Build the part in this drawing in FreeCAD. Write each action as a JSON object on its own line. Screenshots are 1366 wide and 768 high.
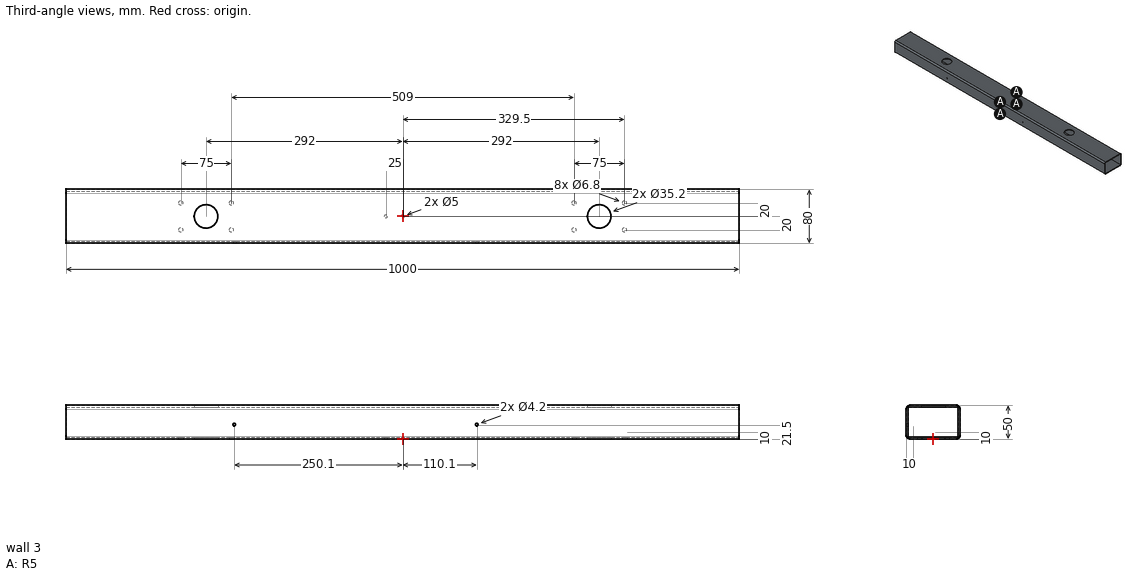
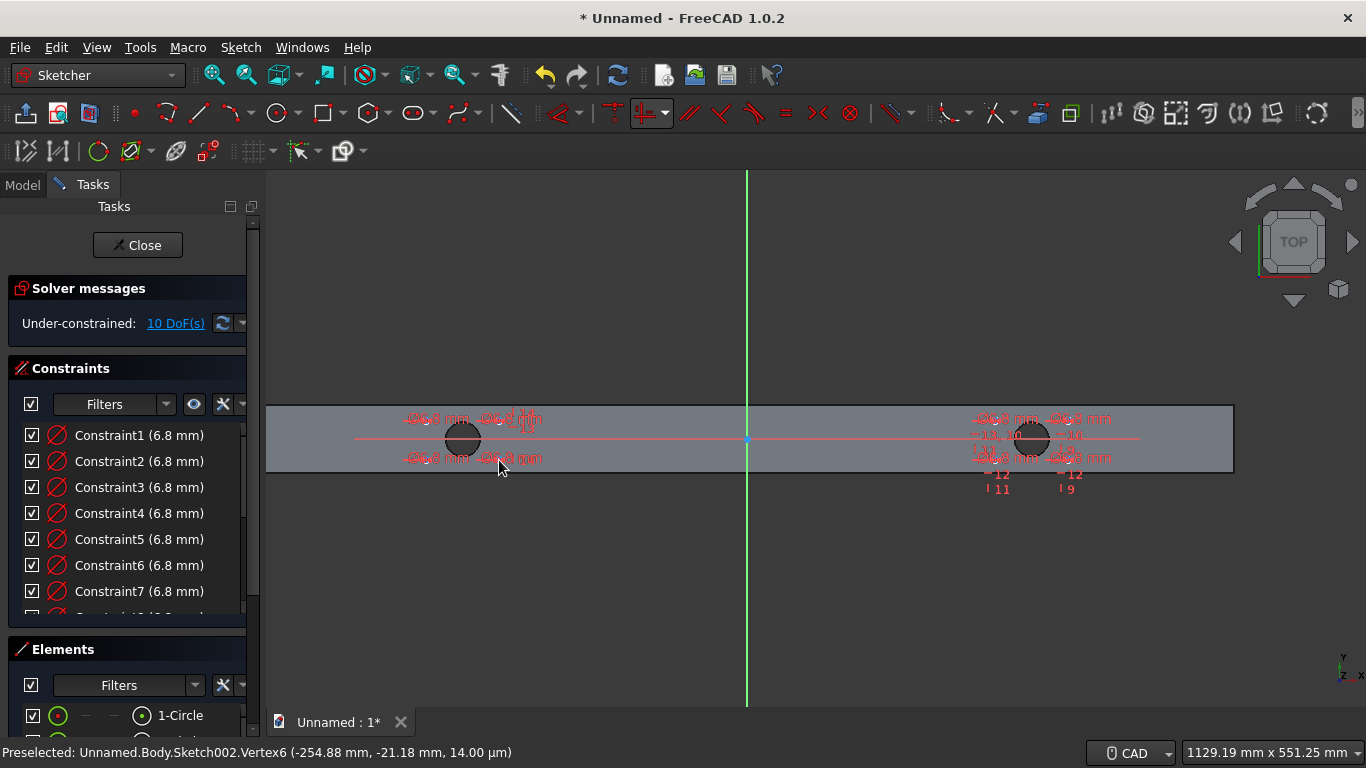
{"action": "left_click", "coordinate": [995, 460]}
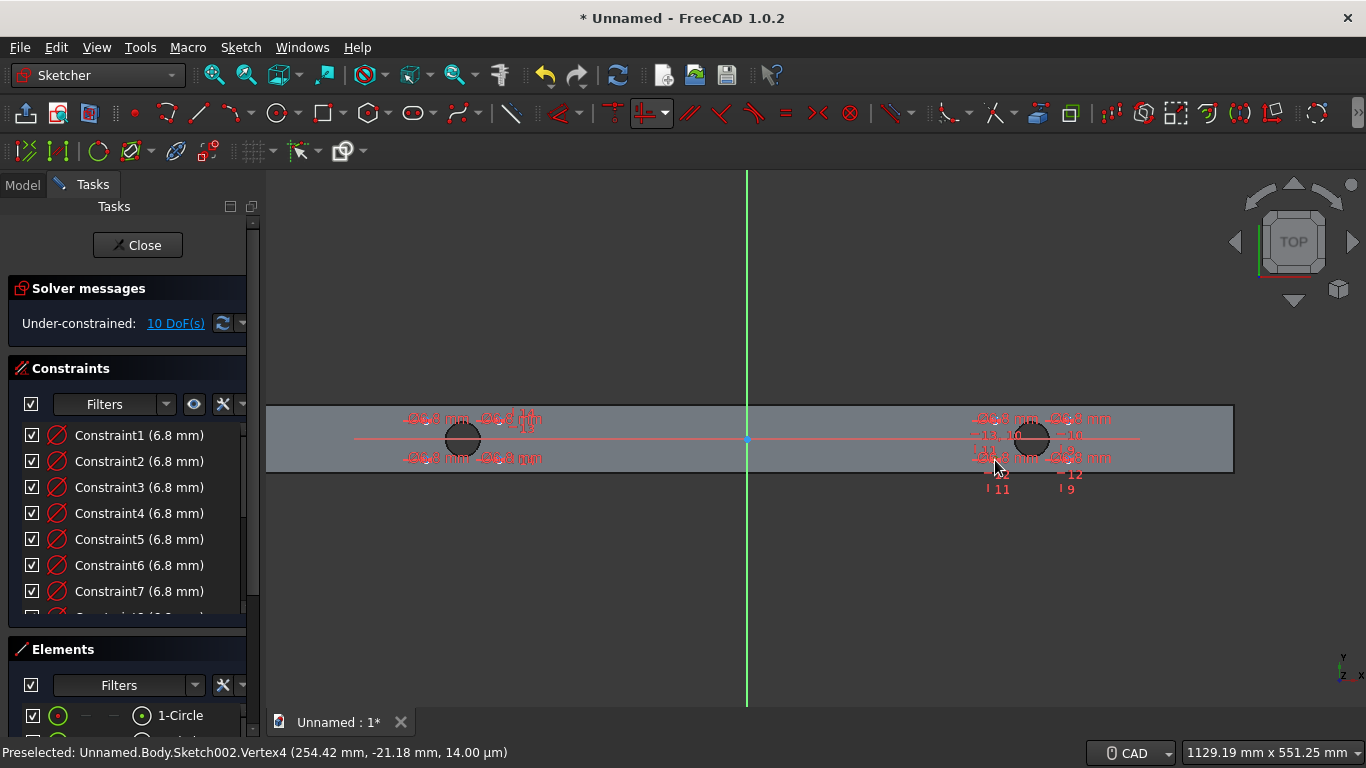
{"action": "left_click", "coordinate": [499, 460]}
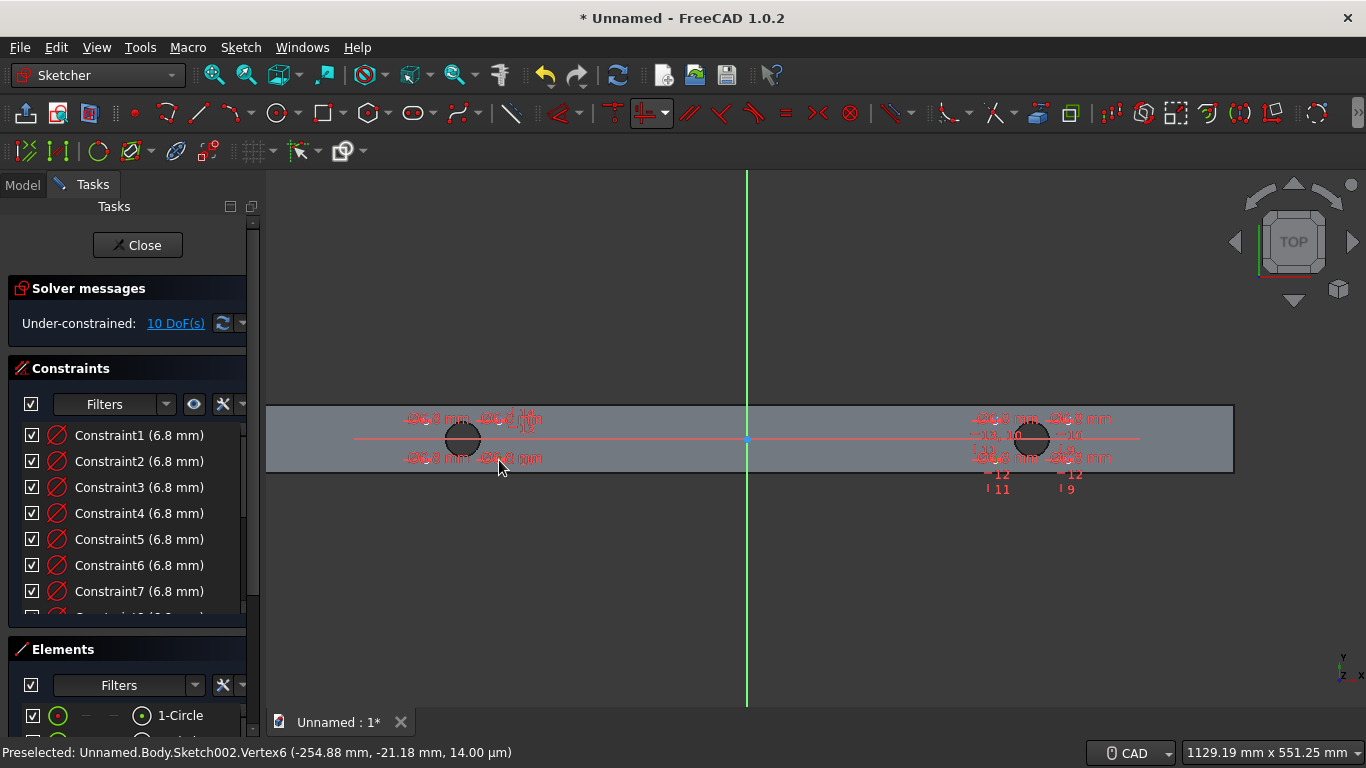
{"action": "left_click", "coordinate": [668, 114]}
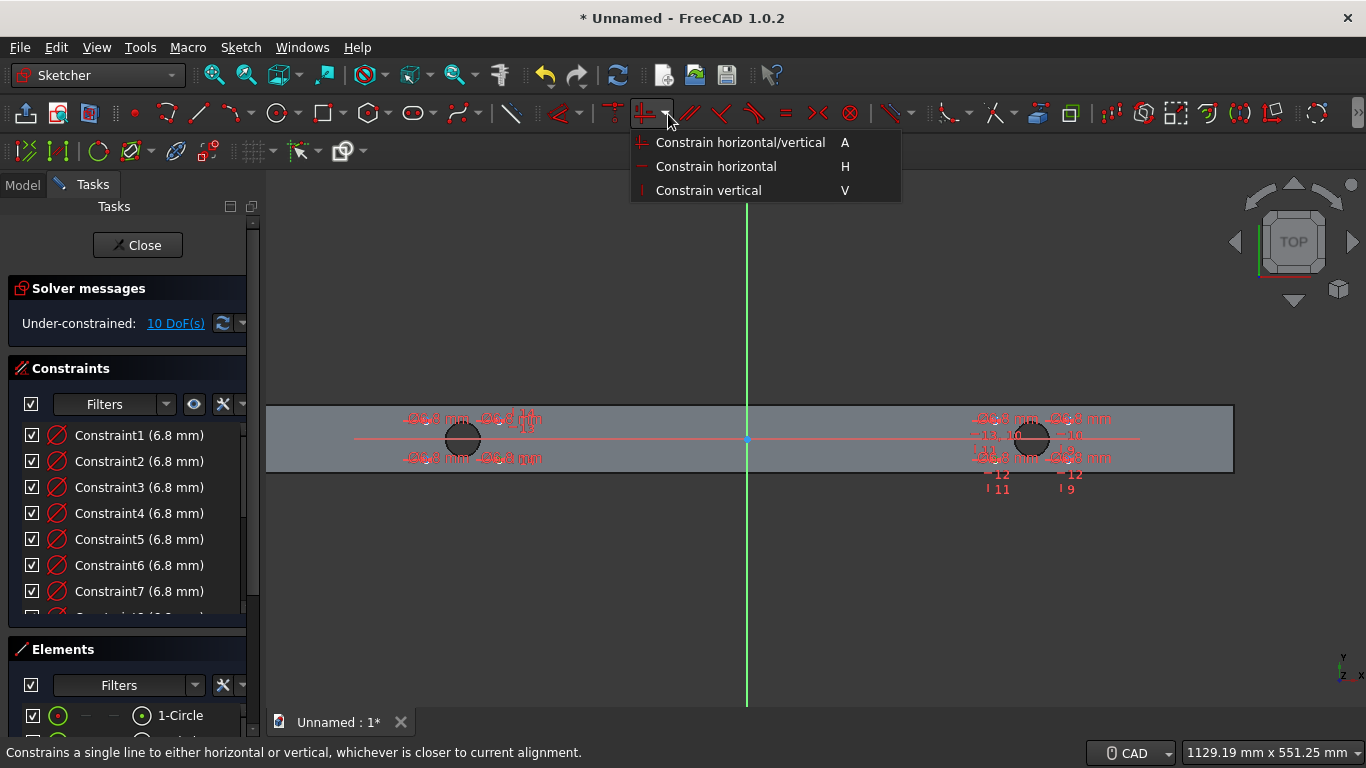
{"action": "left_click", "coordinate": [766, 166]}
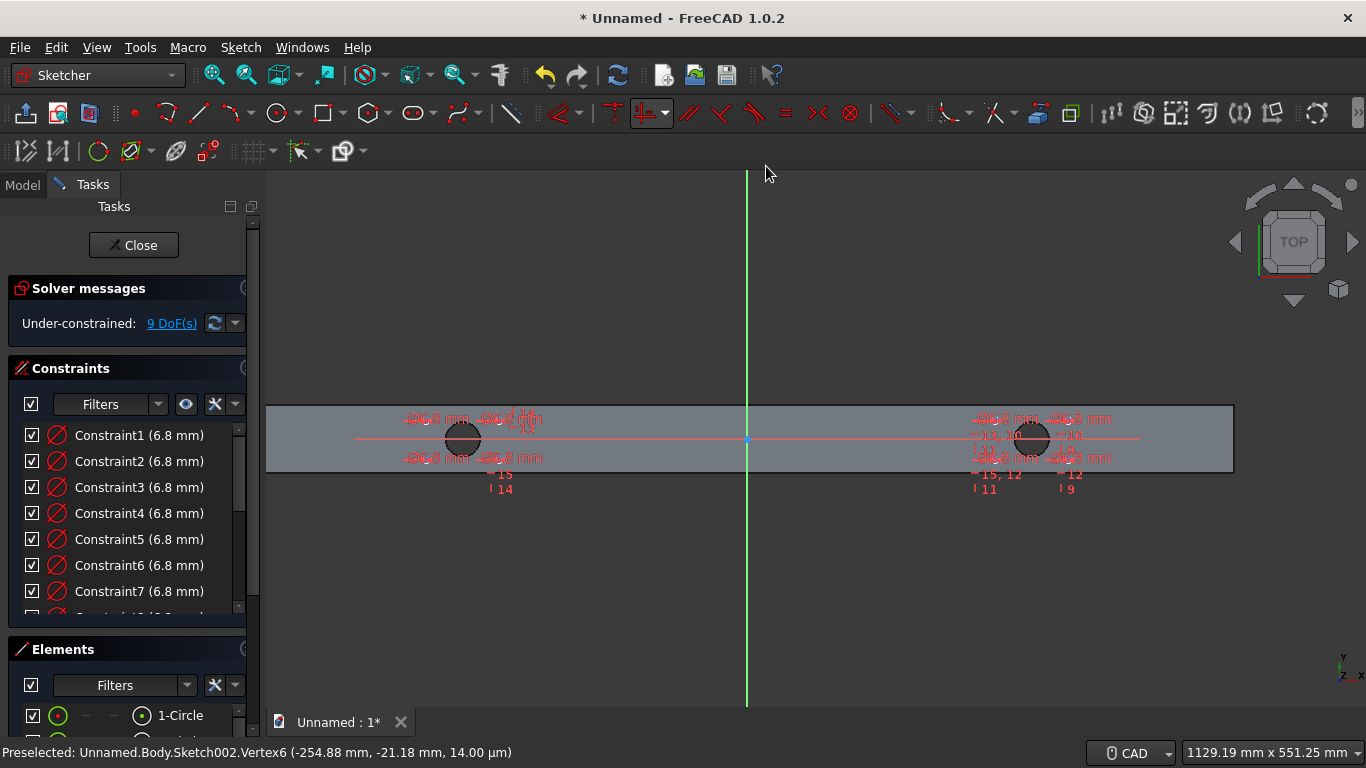
{"action": "left_click", "coordinate": [499, 421]}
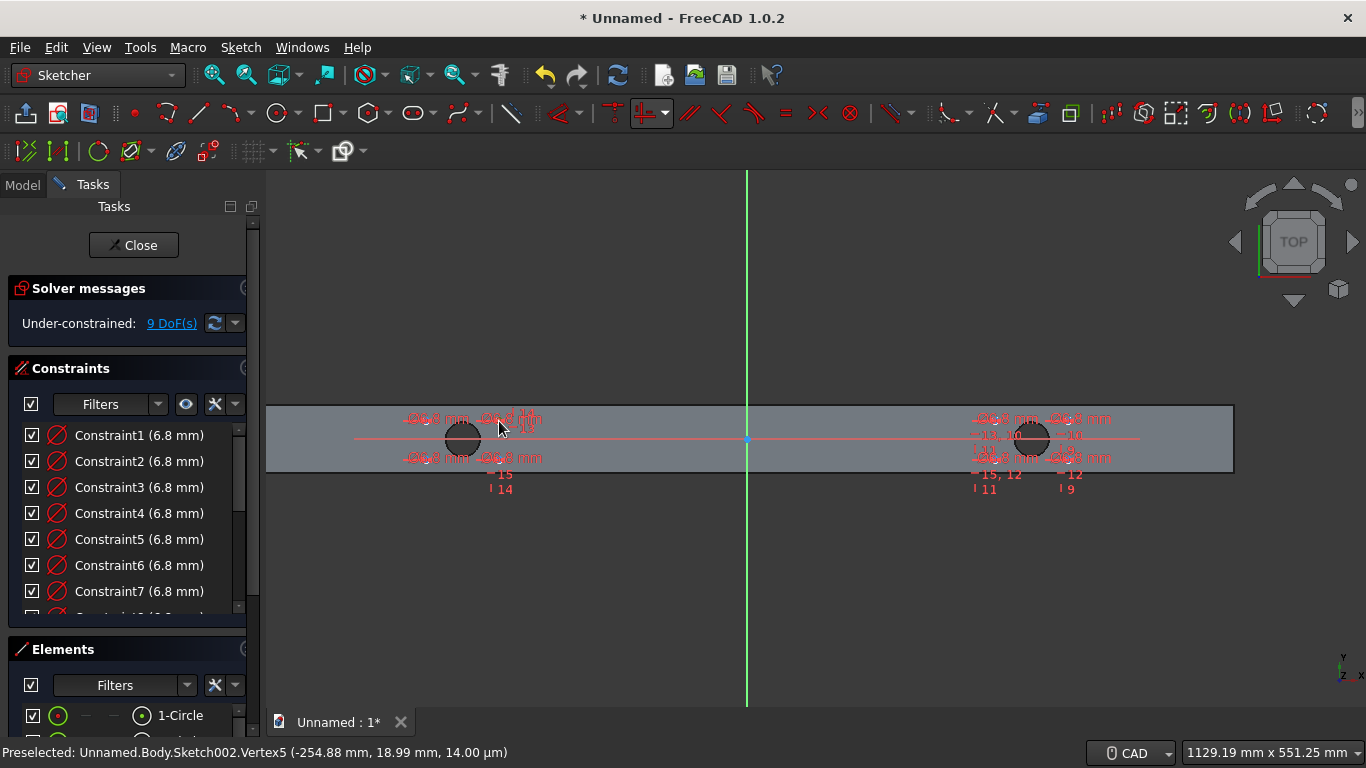
{"action": "left_click", "coordinate": [426, 421]}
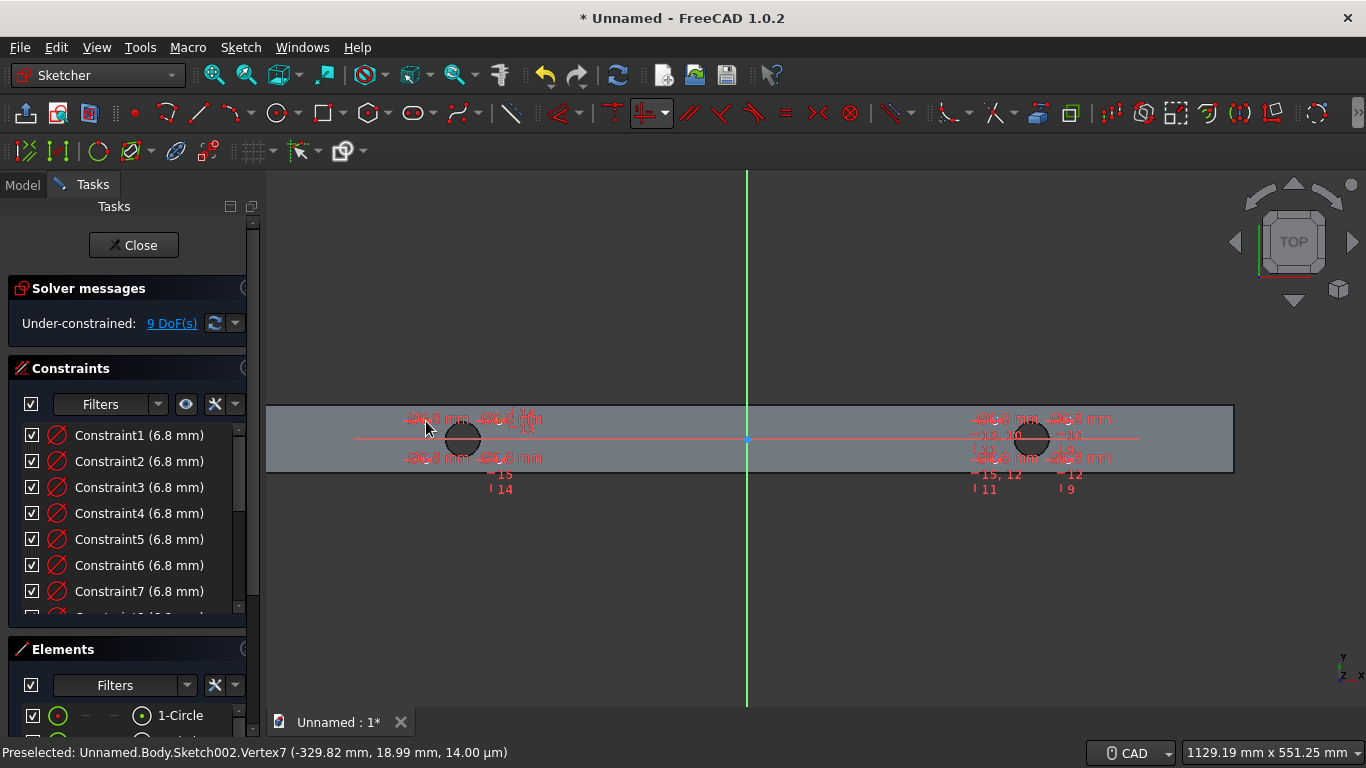
{"action": "key", "text": "h"}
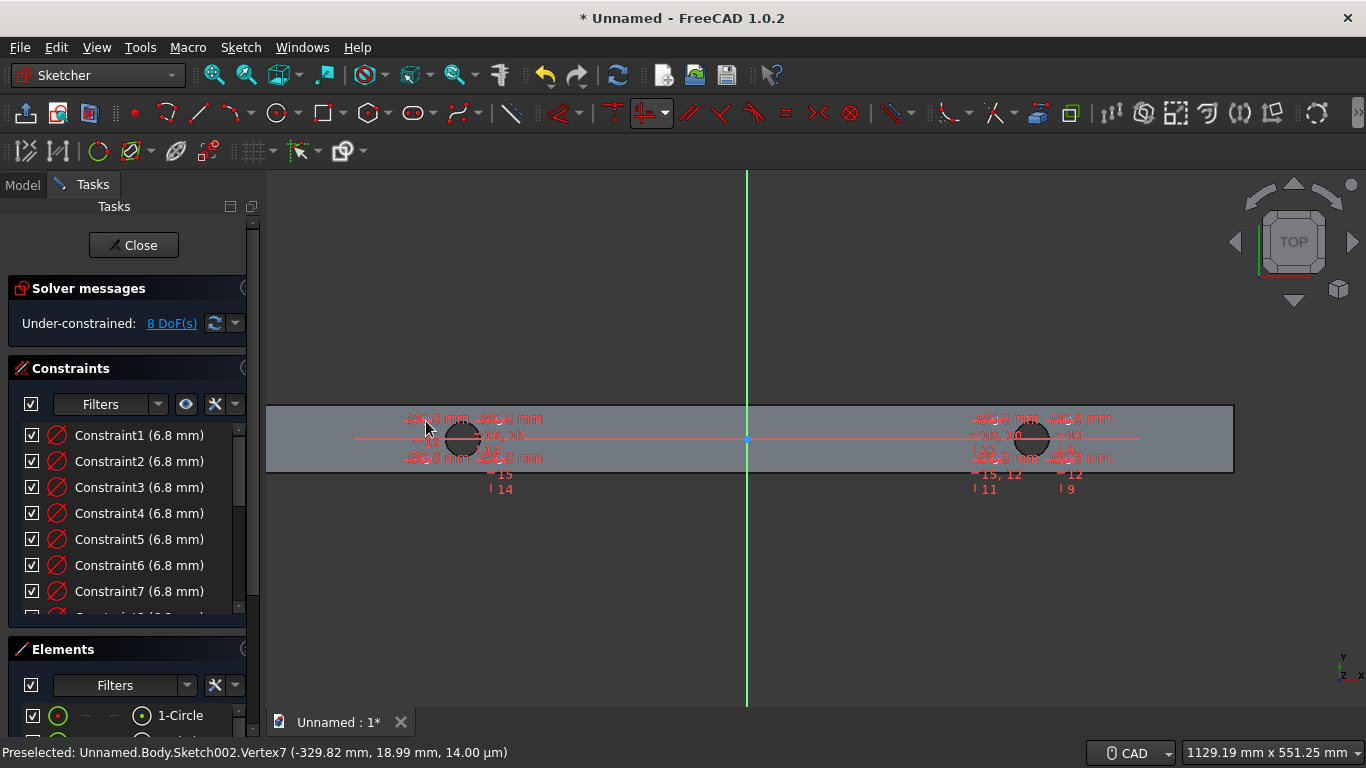
{"action": "left_click", "coordinate": [426, 421]}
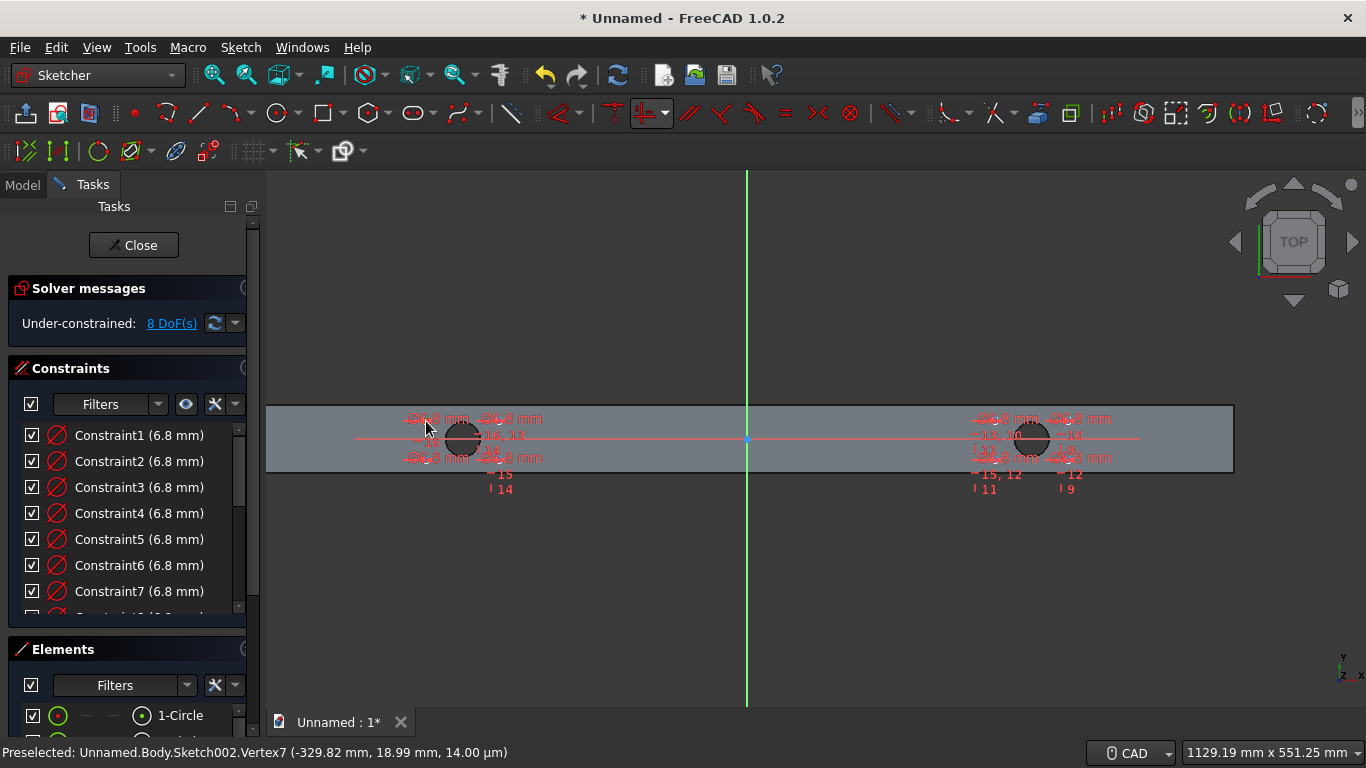
{"action": "left_click", "coordinate": [426, 460]}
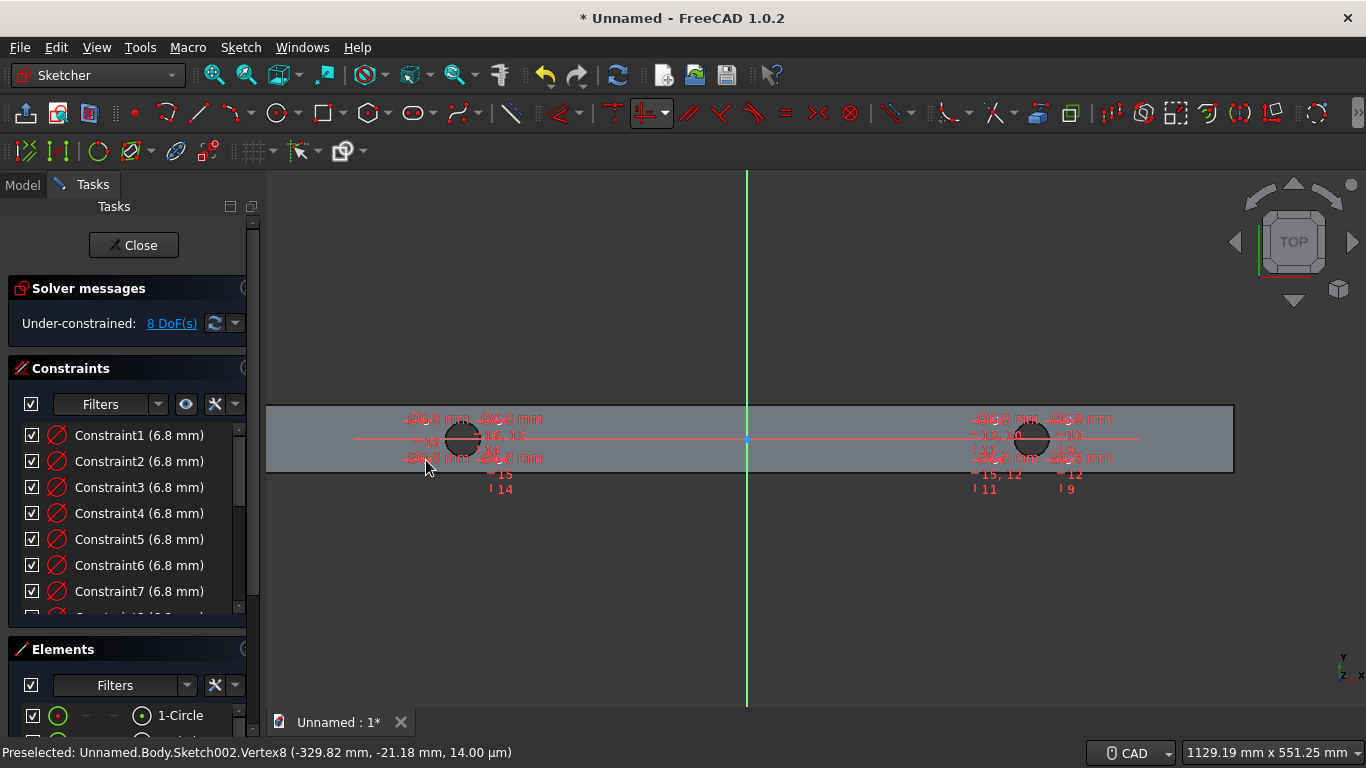
{"action": "left_click", "coordinate": [668, 114]}